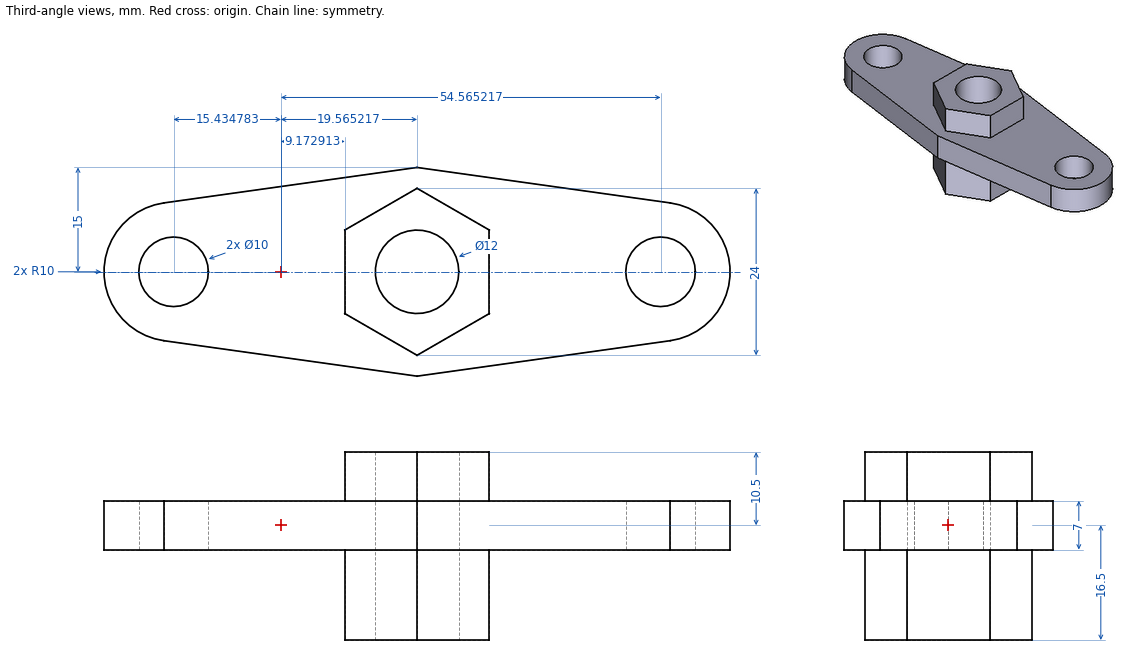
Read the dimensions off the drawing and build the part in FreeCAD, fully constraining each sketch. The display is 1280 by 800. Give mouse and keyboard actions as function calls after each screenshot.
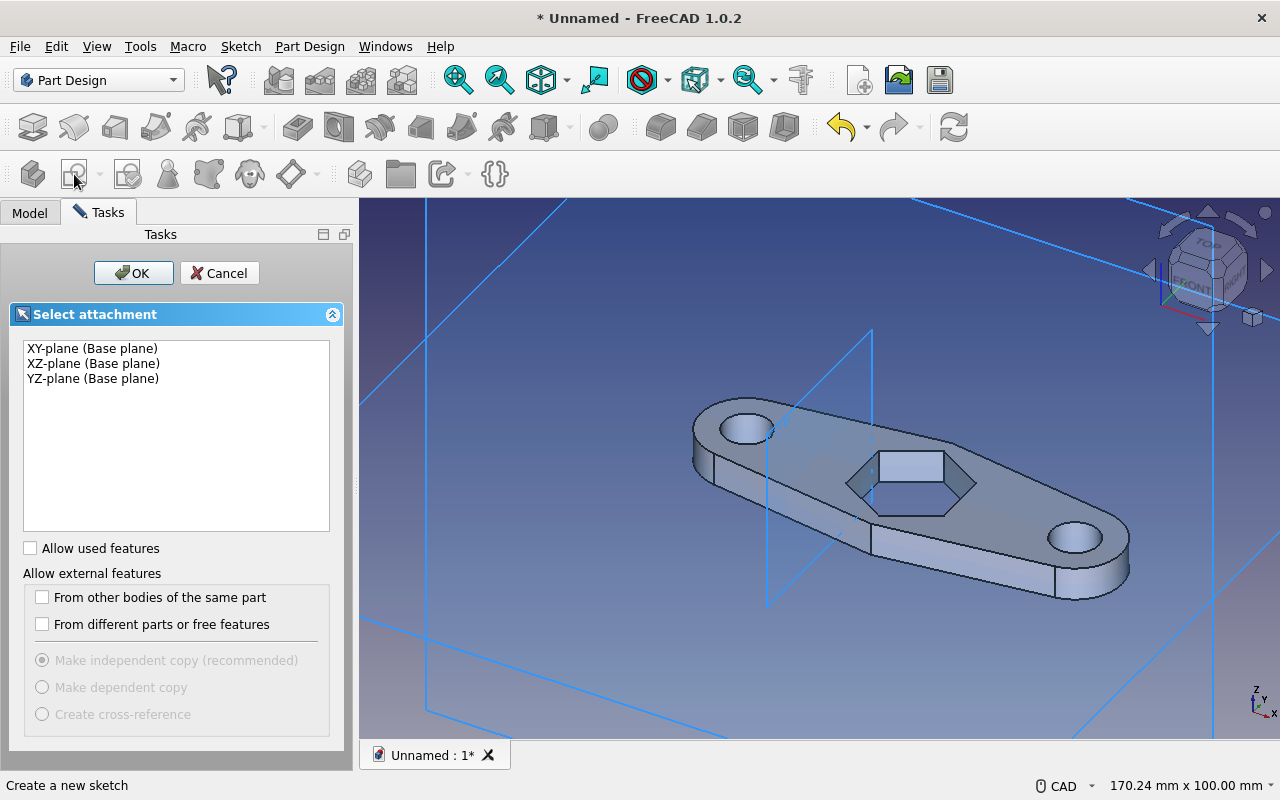
click(84, 348)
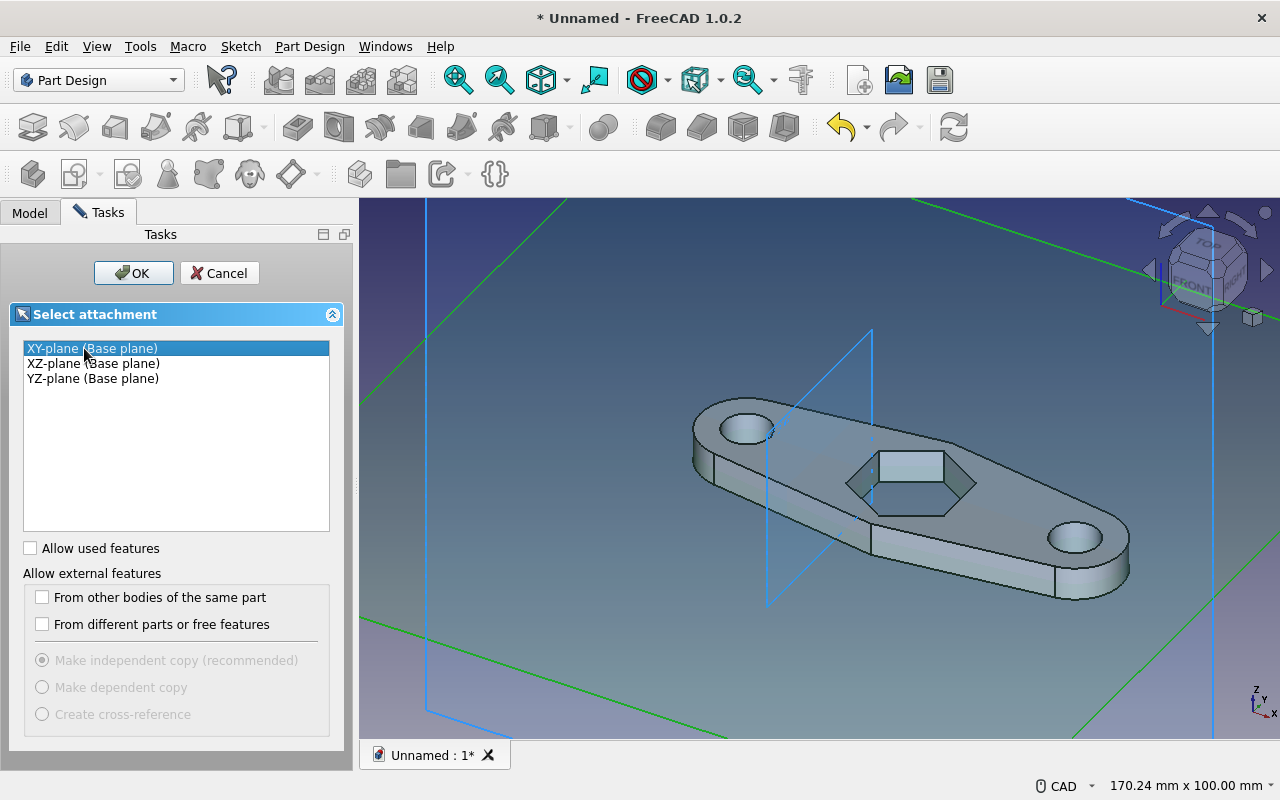
click(134, 273)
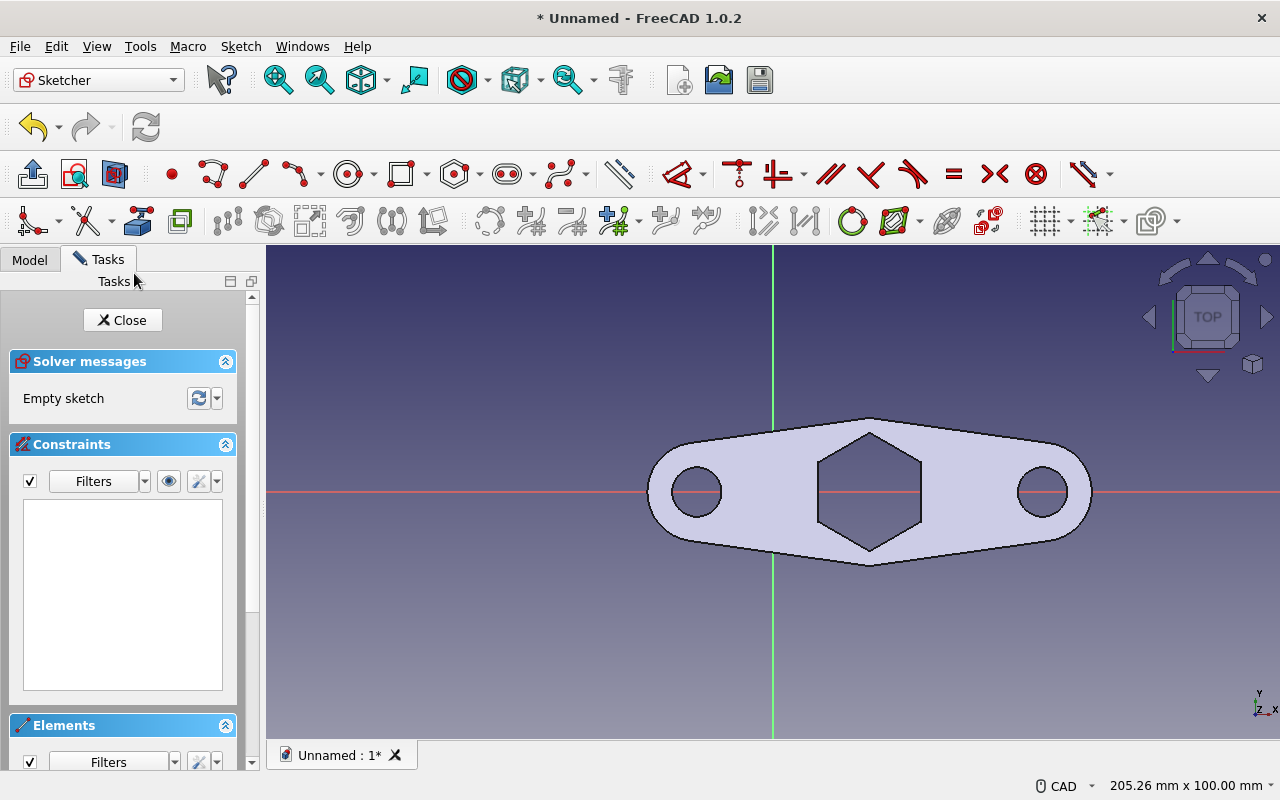
click(115, 174)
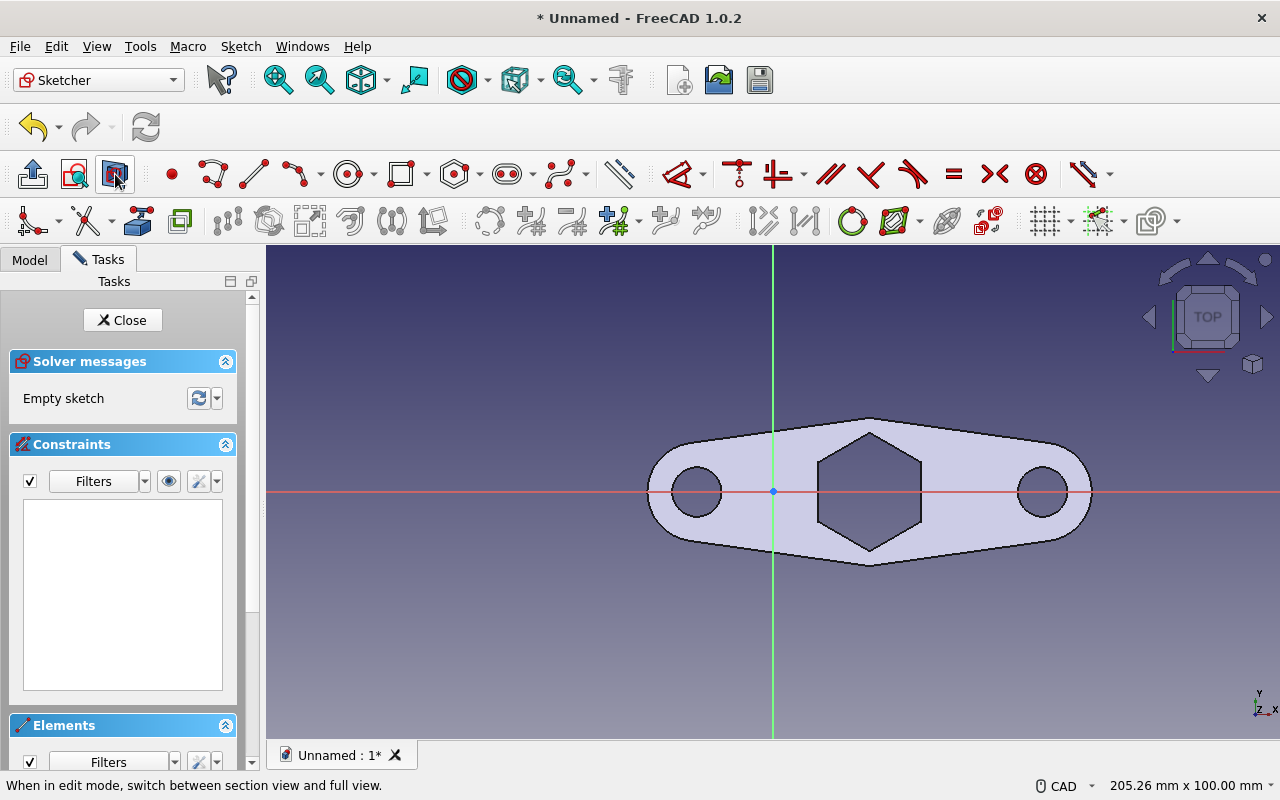
scroll(930, 492, up, 5)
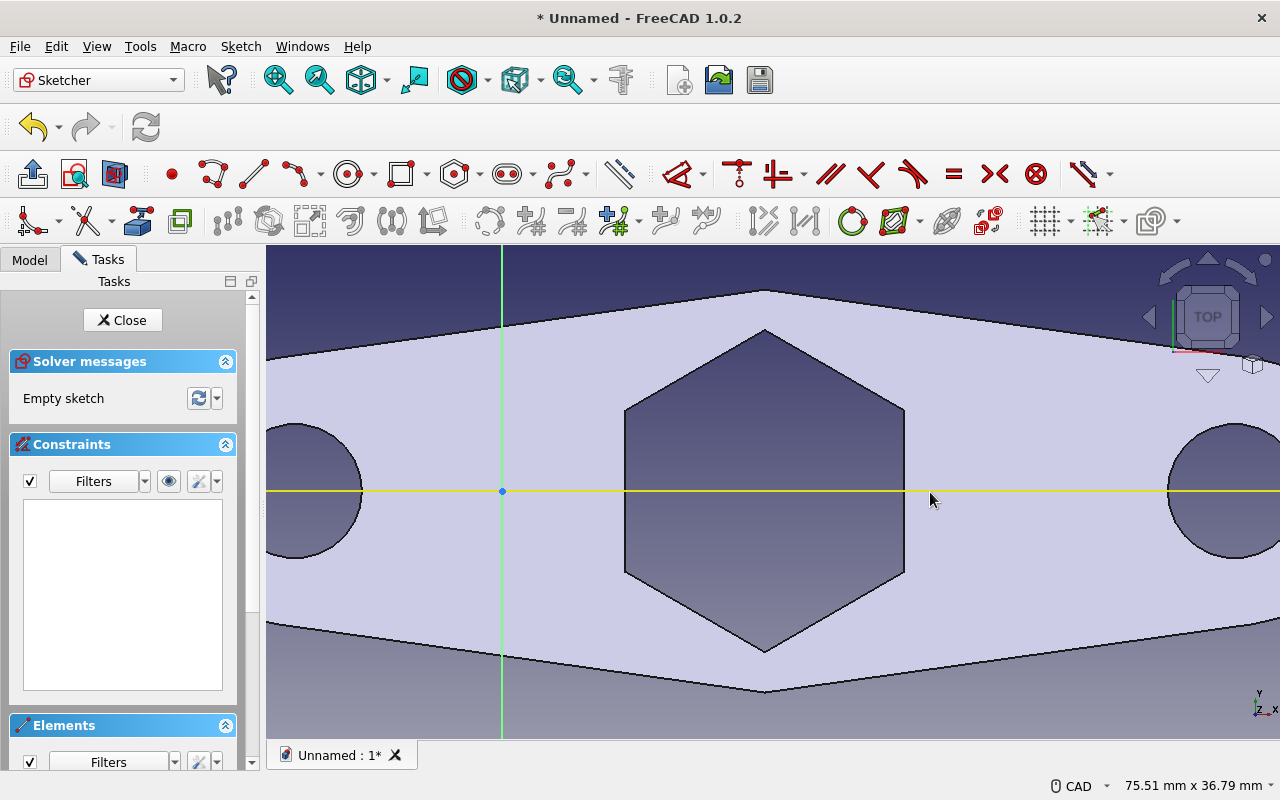
click(454, 174)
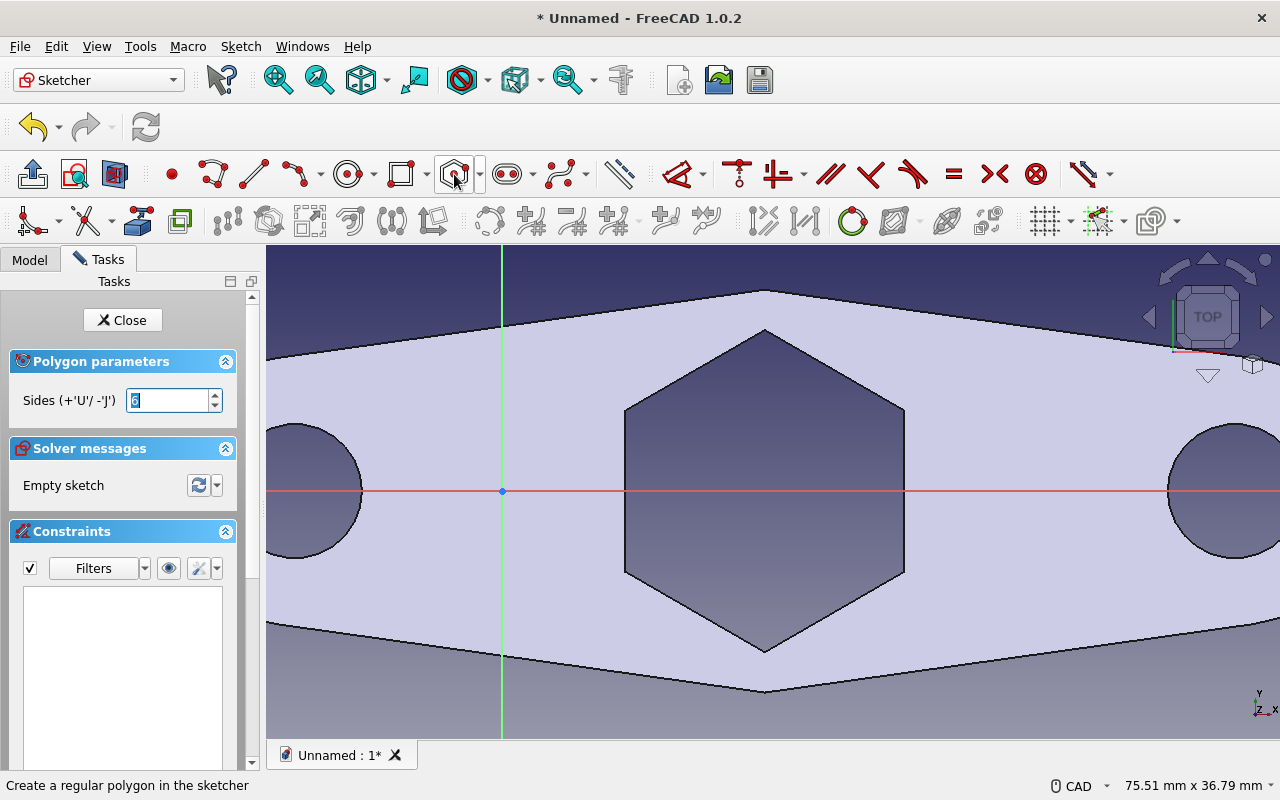
click(765, 491)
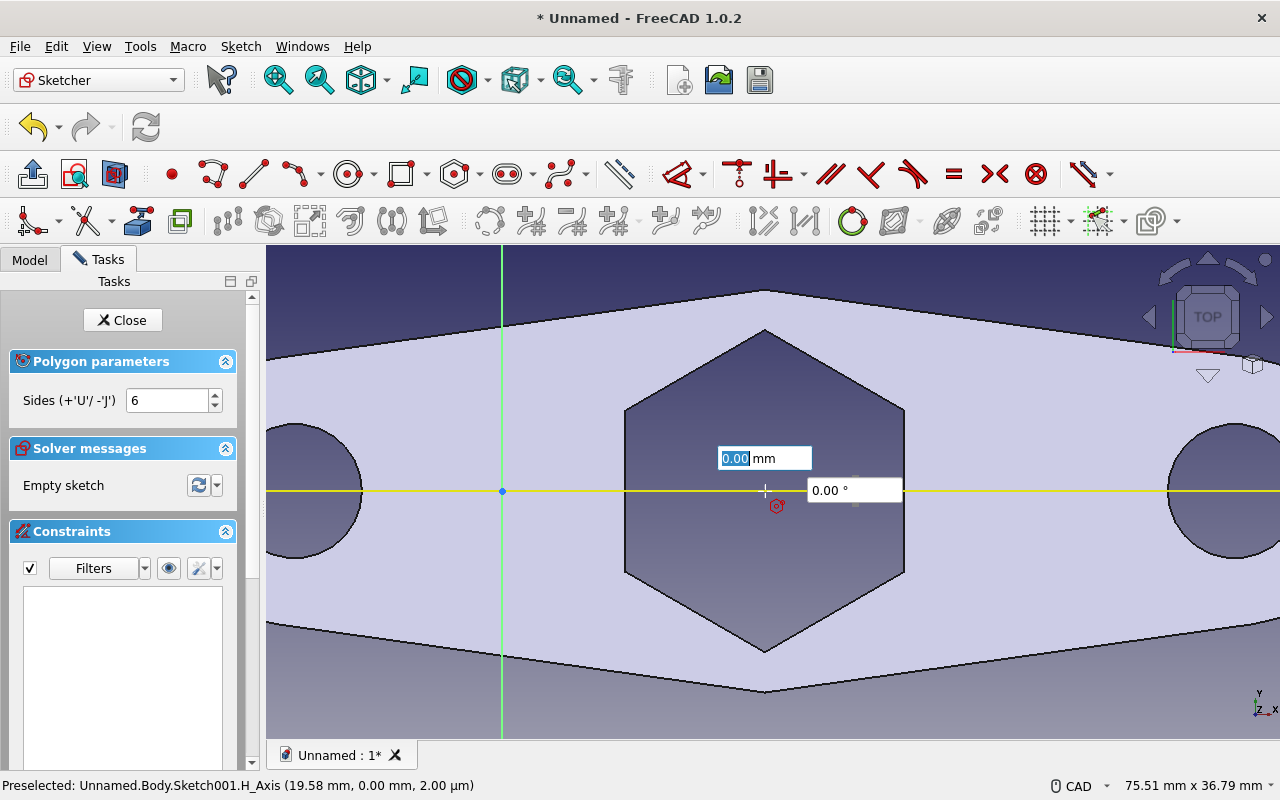
click(765, 652)
right_click(765, 652)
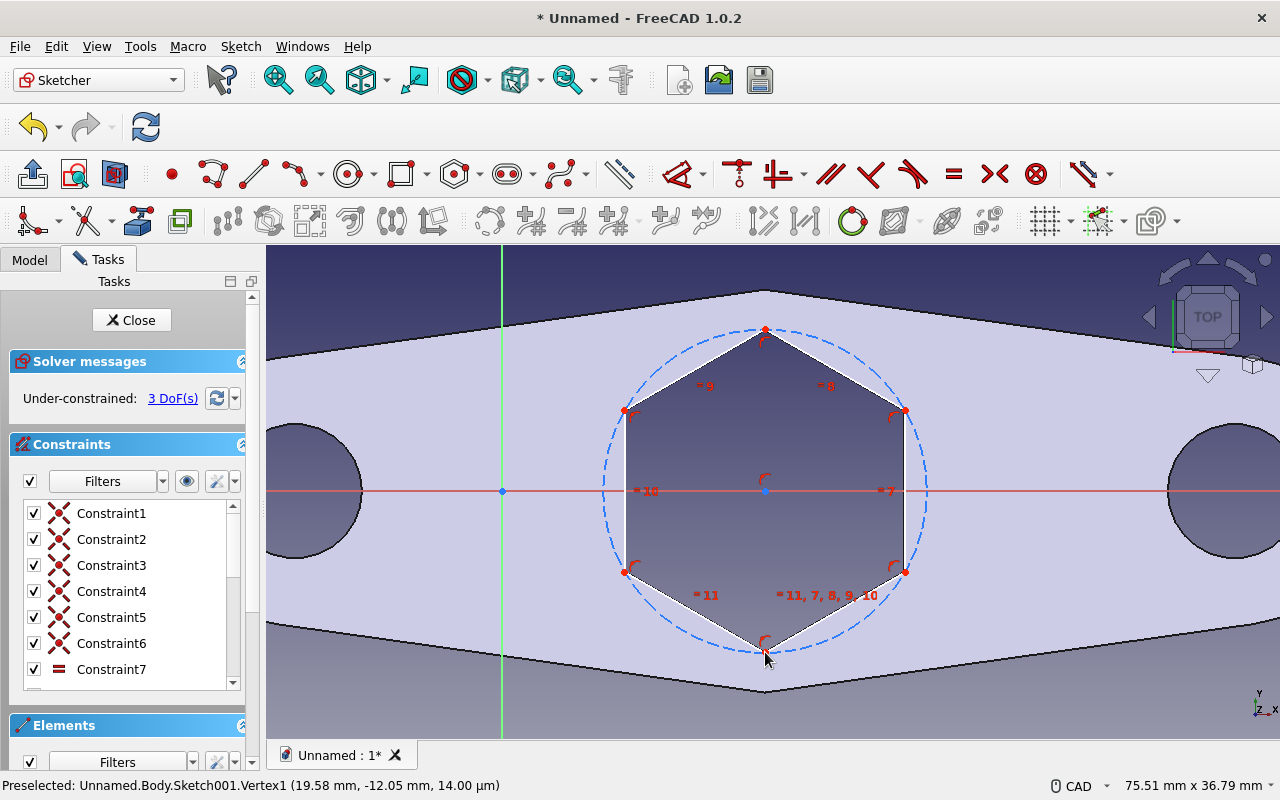
click(905, 524)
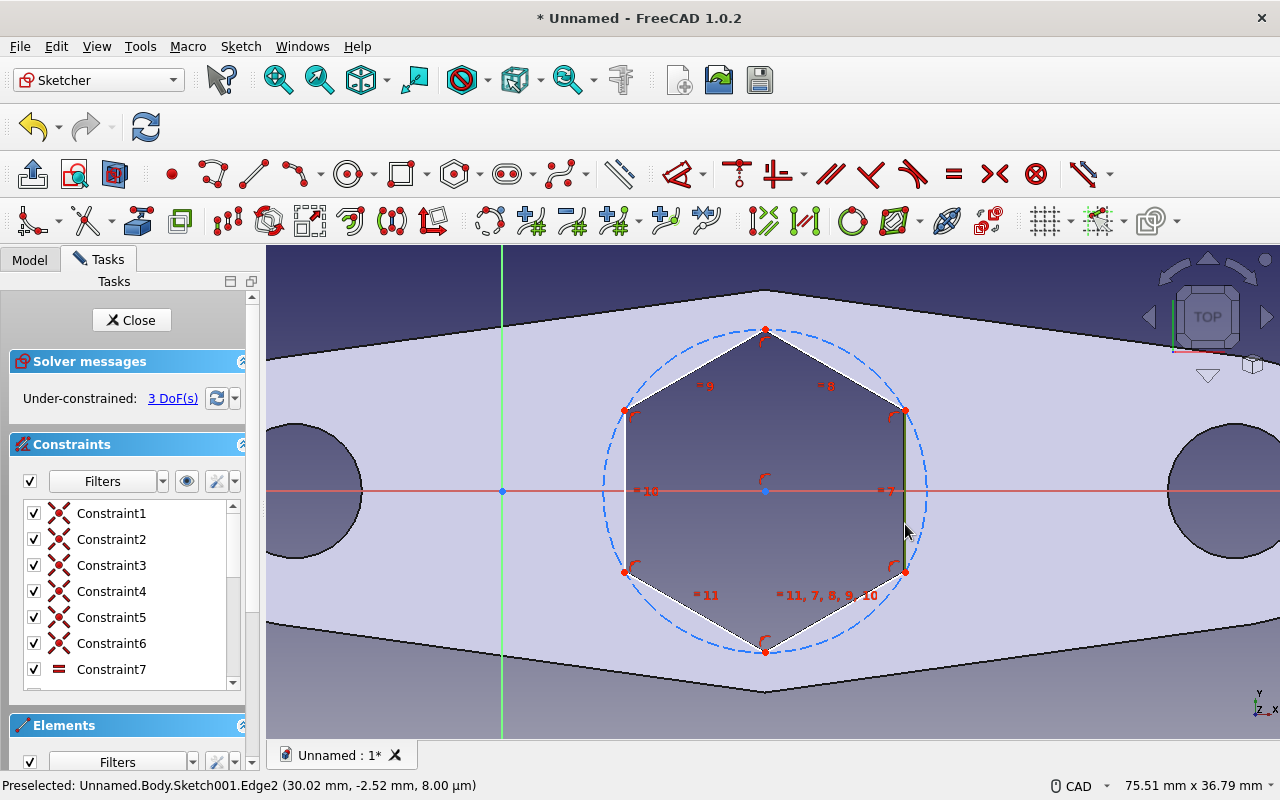
click(804, 174)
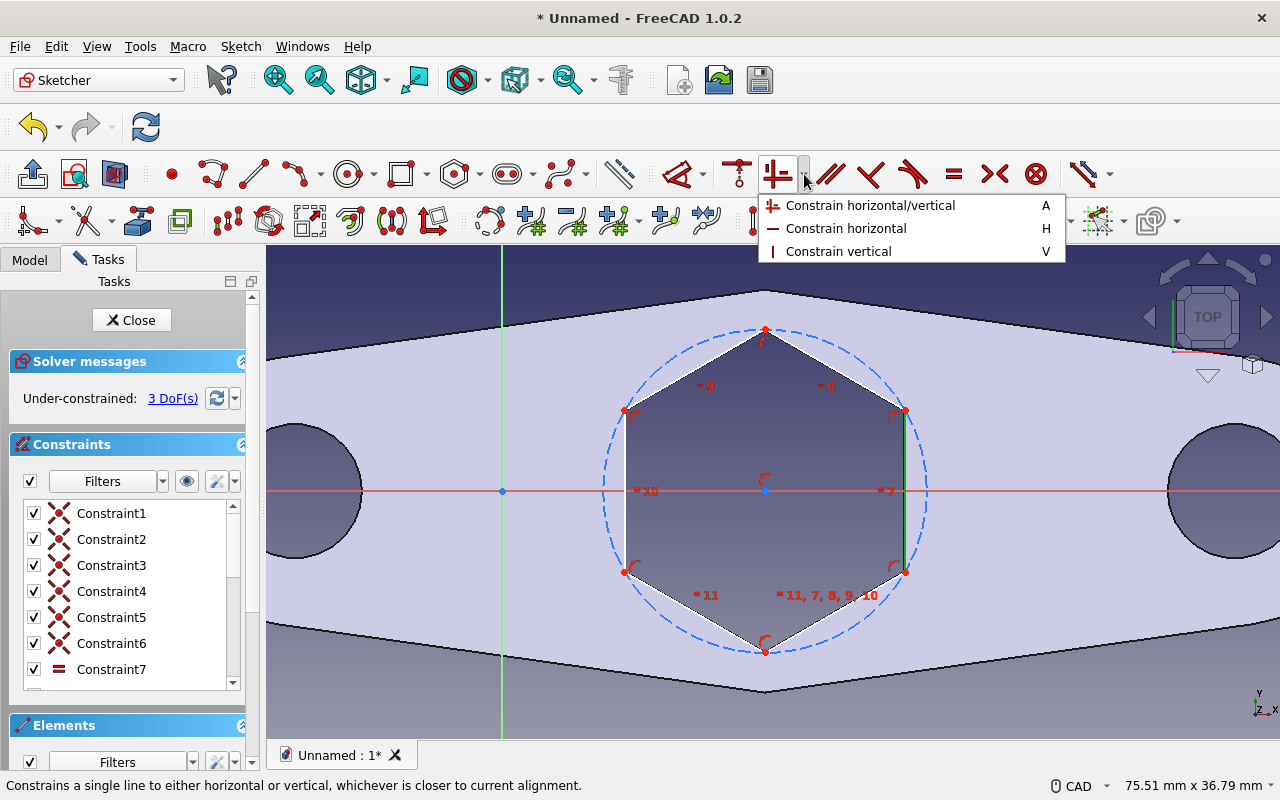
click(912, 252)